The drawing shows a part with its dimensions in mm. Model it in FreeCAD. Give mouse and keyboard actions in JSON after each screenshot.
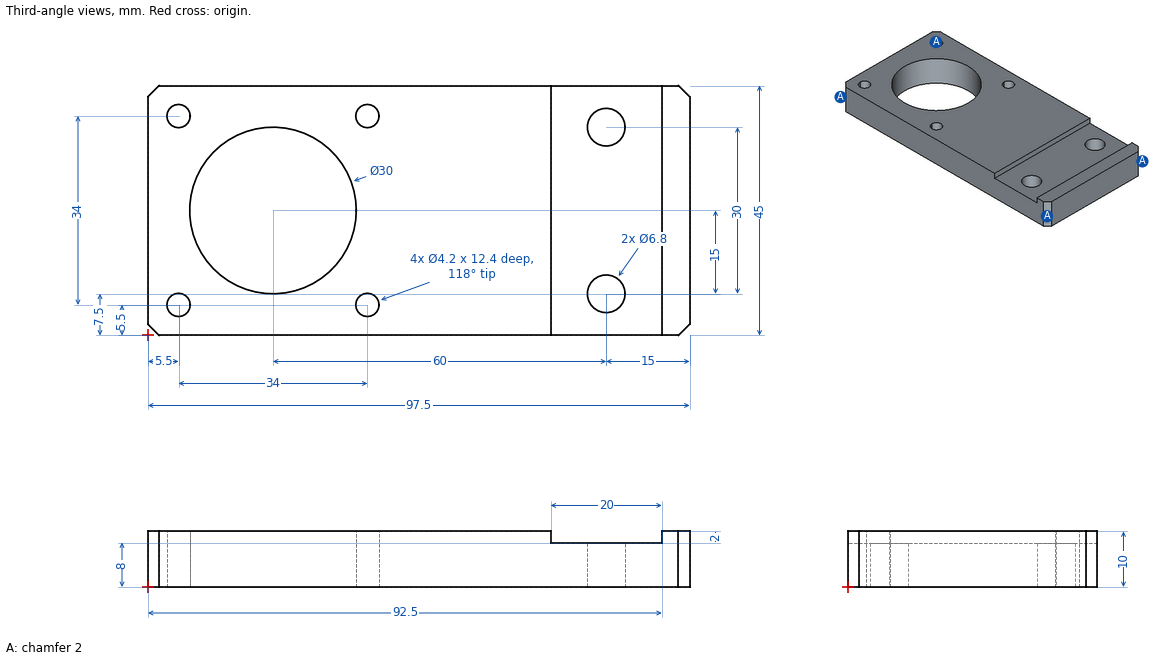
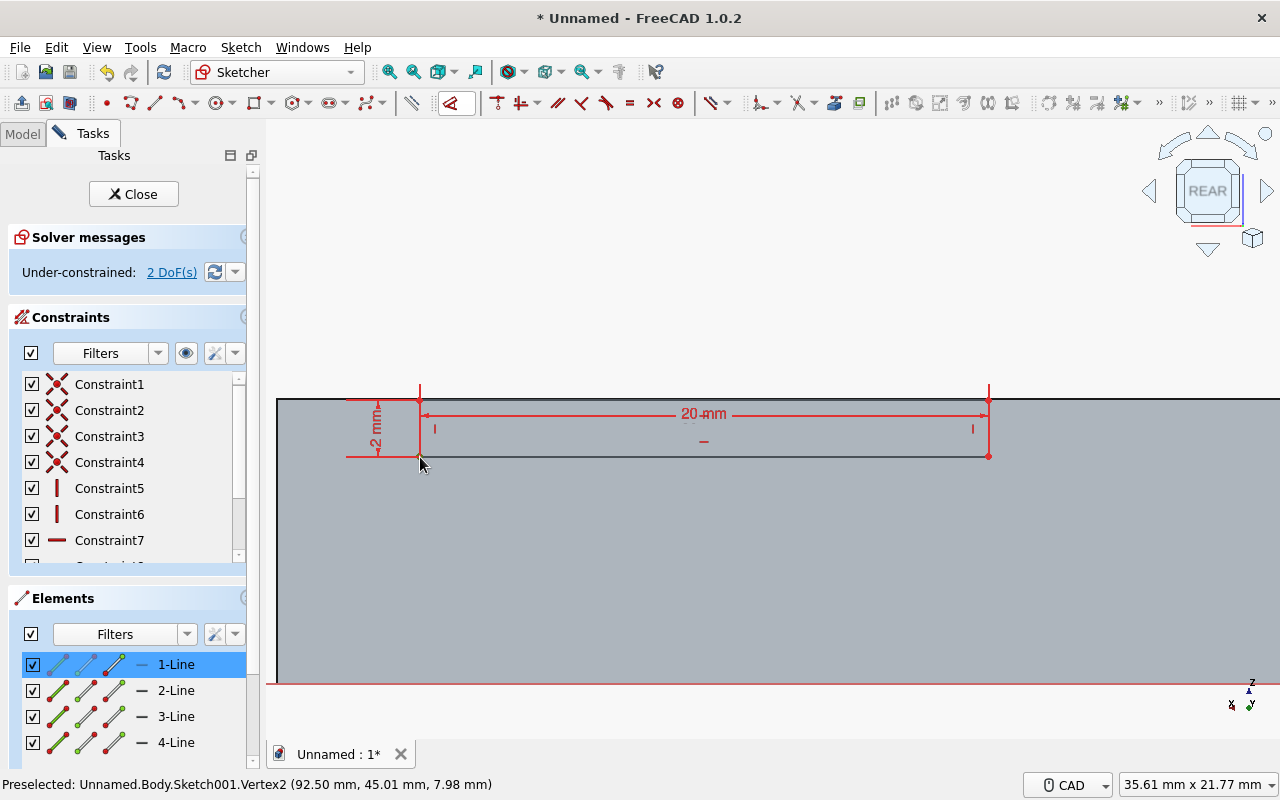
{"action": "key", "text": "i"}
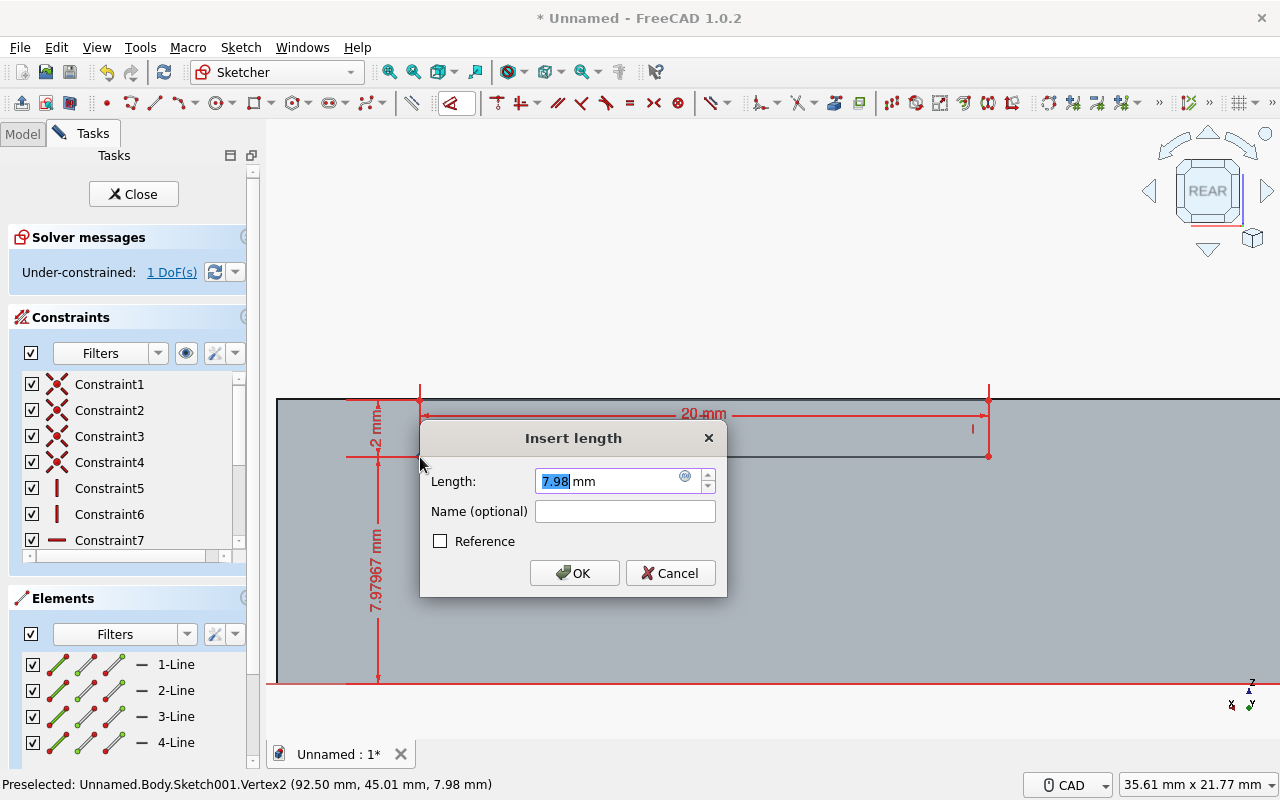
{"action": "type", "text": "8"}
{"action": "key", "text": "Return"}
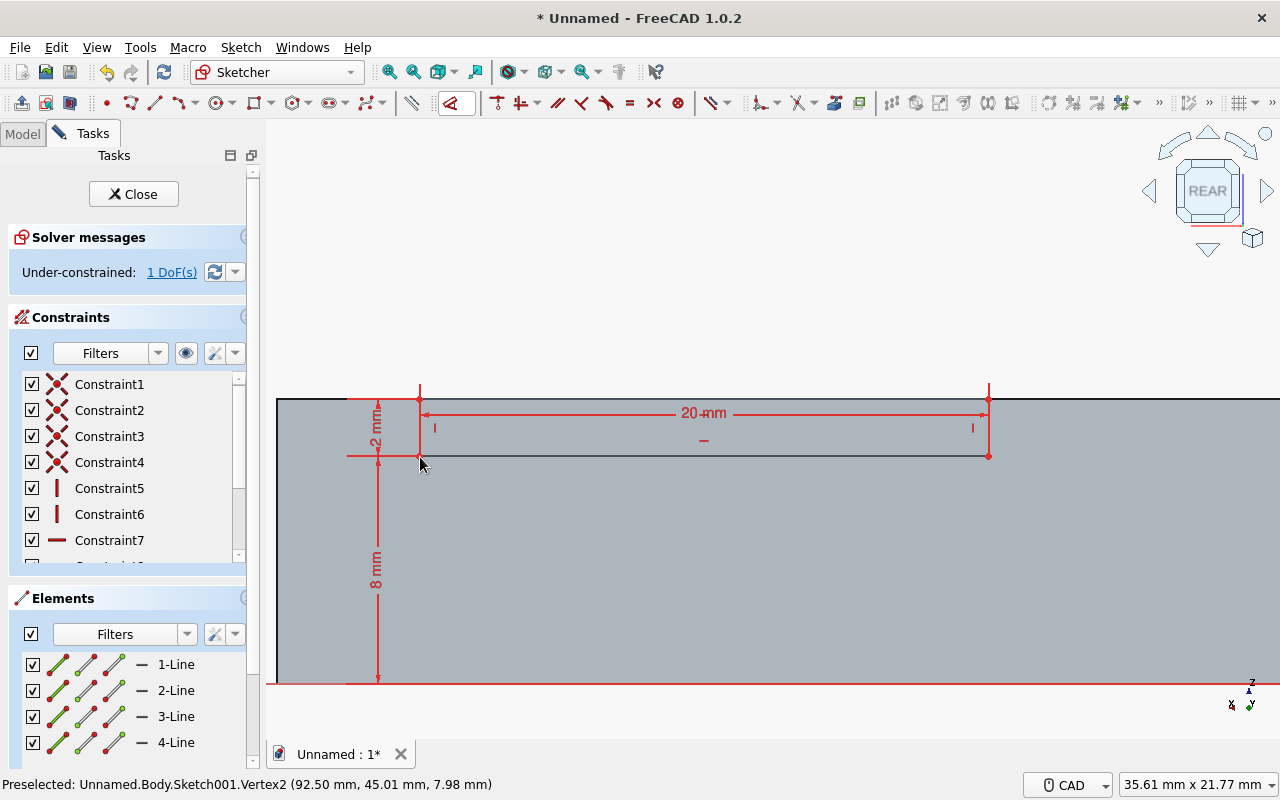
{"action": "left_click", "coordinate": [420, 399]}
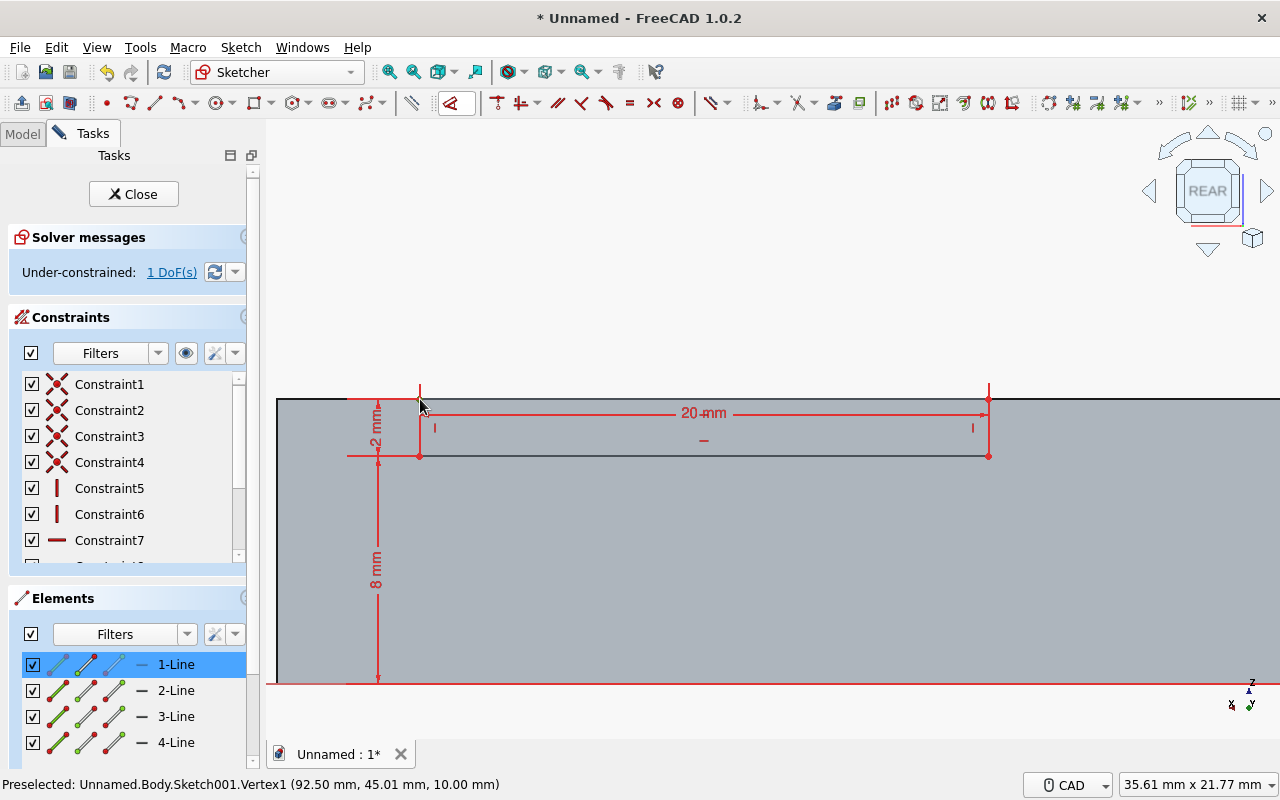
{"action": "left_click", "coordinate": [470, 104]}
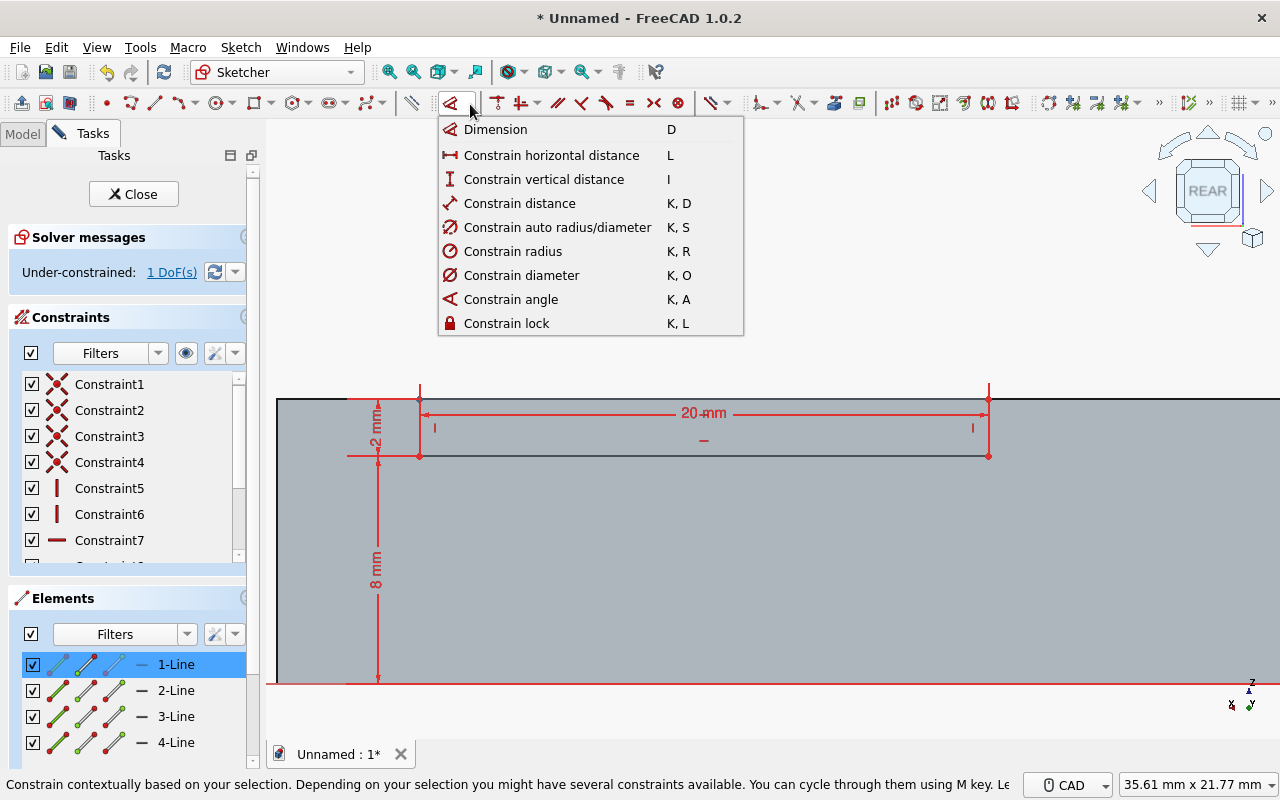
{"action": "left_click", "coordinate": [591, 155]}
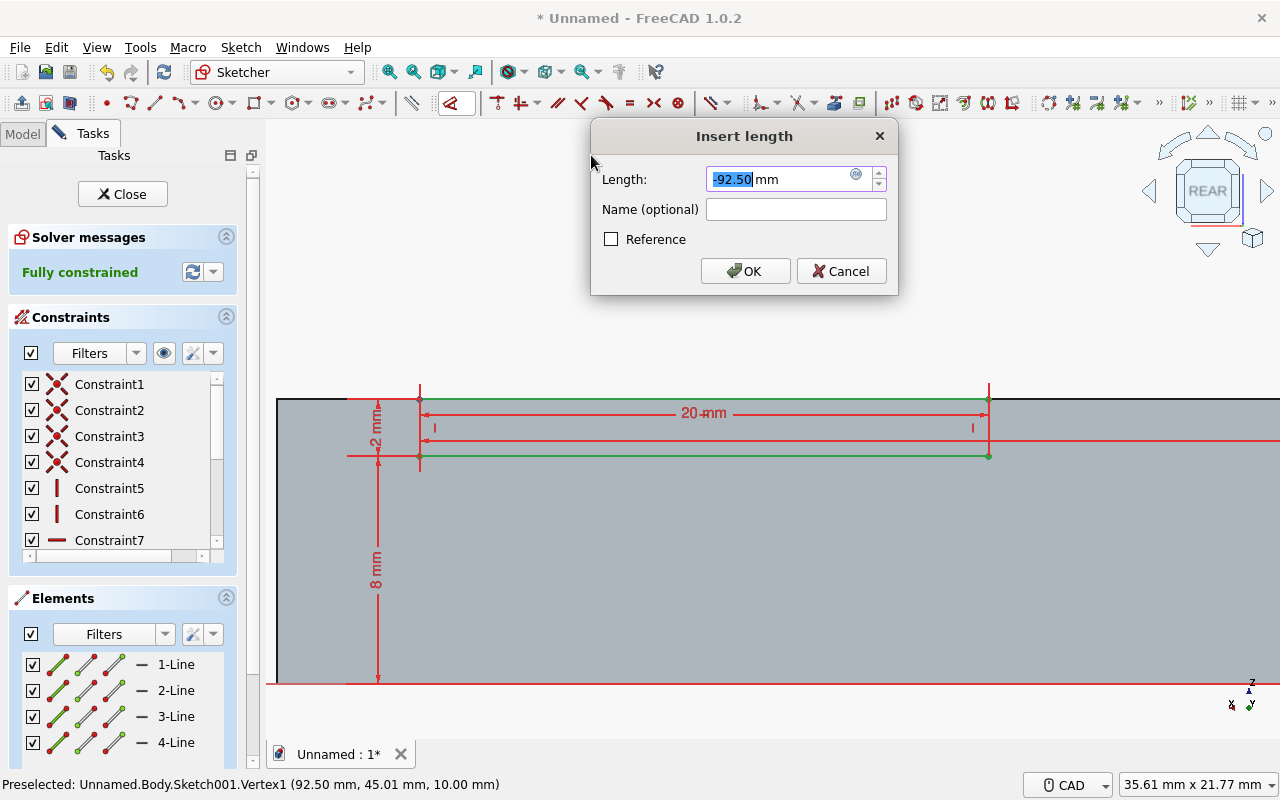
{"action": "type", "text": "-92.5"}
{"action": "key", "text": "Return"}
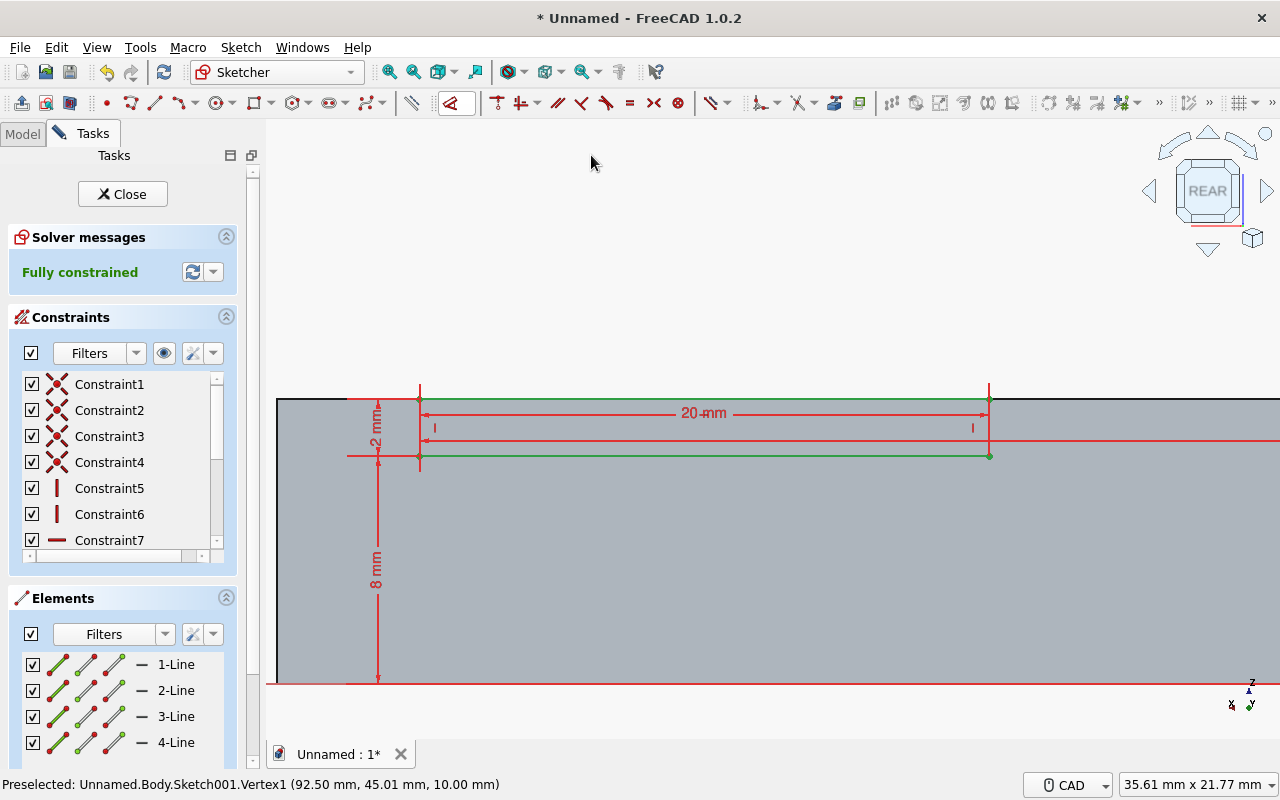
{"action": "left_click", "coordinate": [123, 194]}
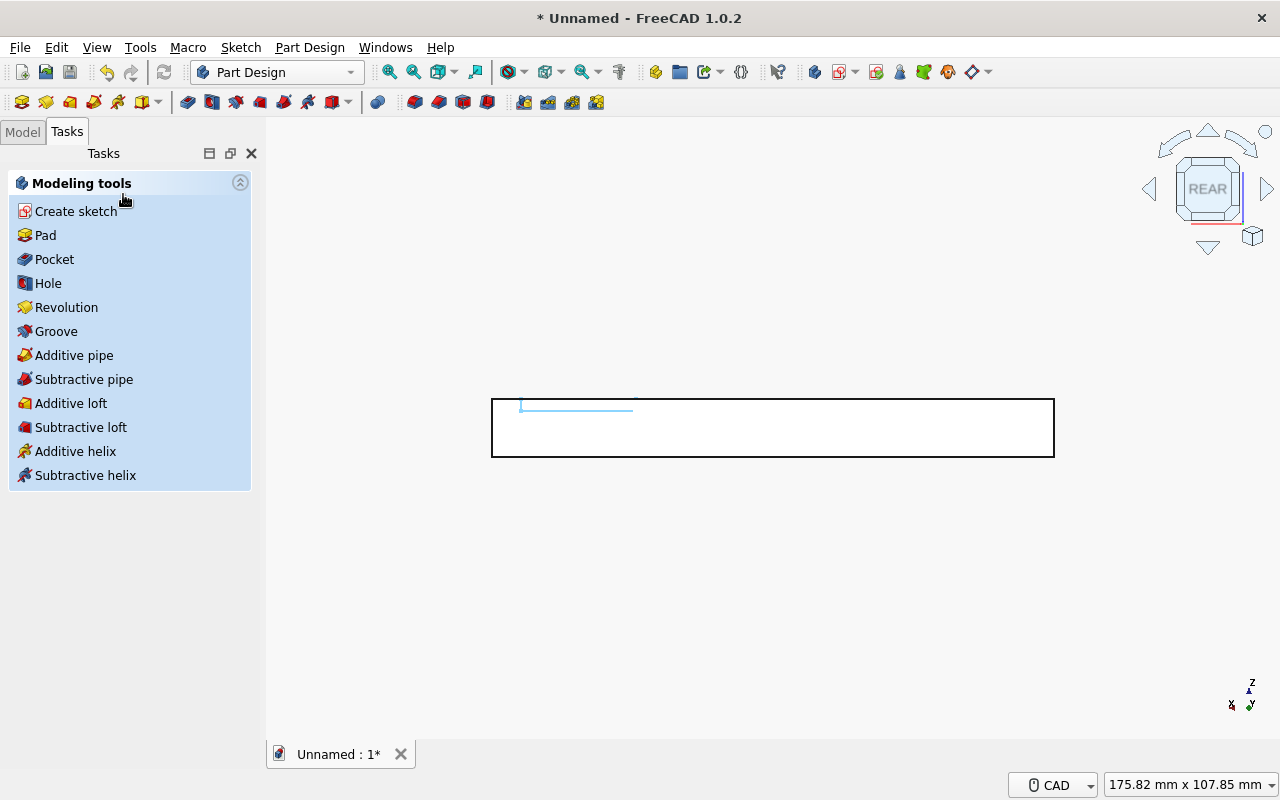
{"action": "left_click", "coordinate": [188, 102]}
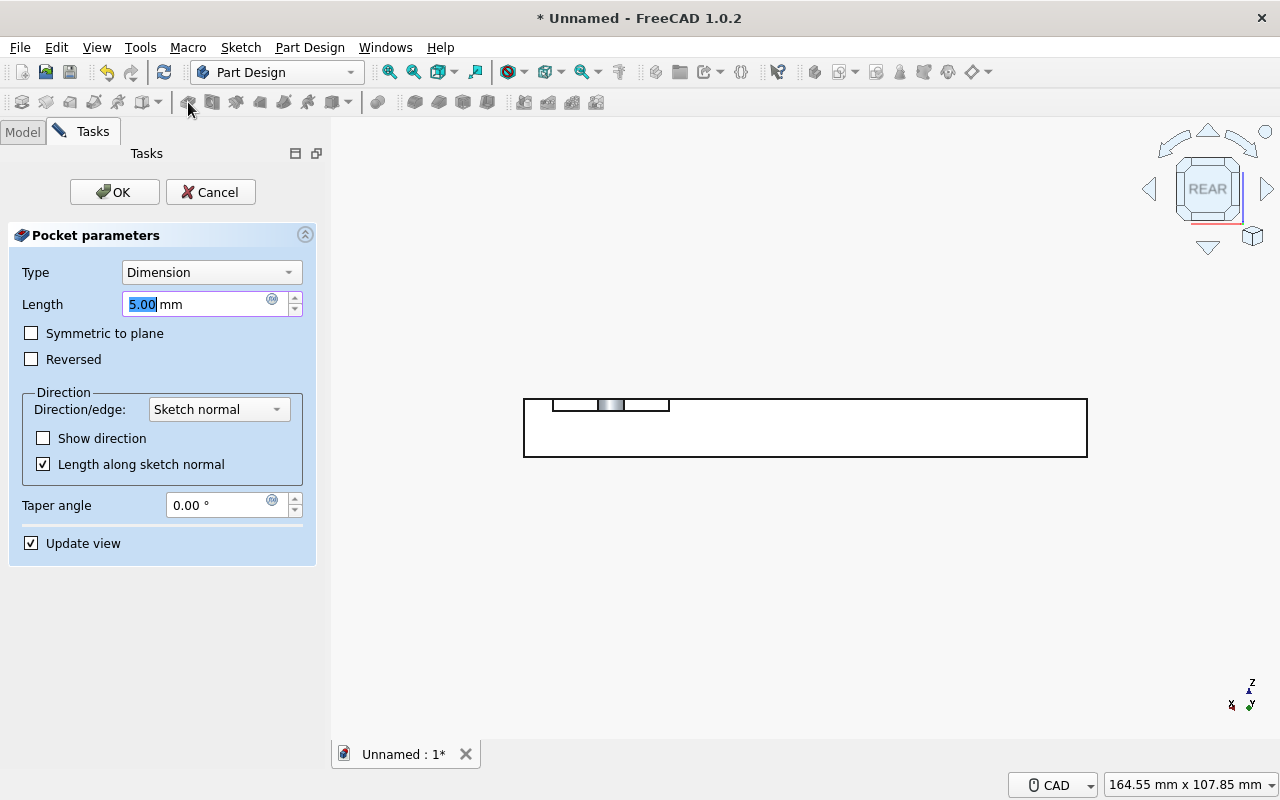
{"action": "left_click", "coordinate": [212, 272]}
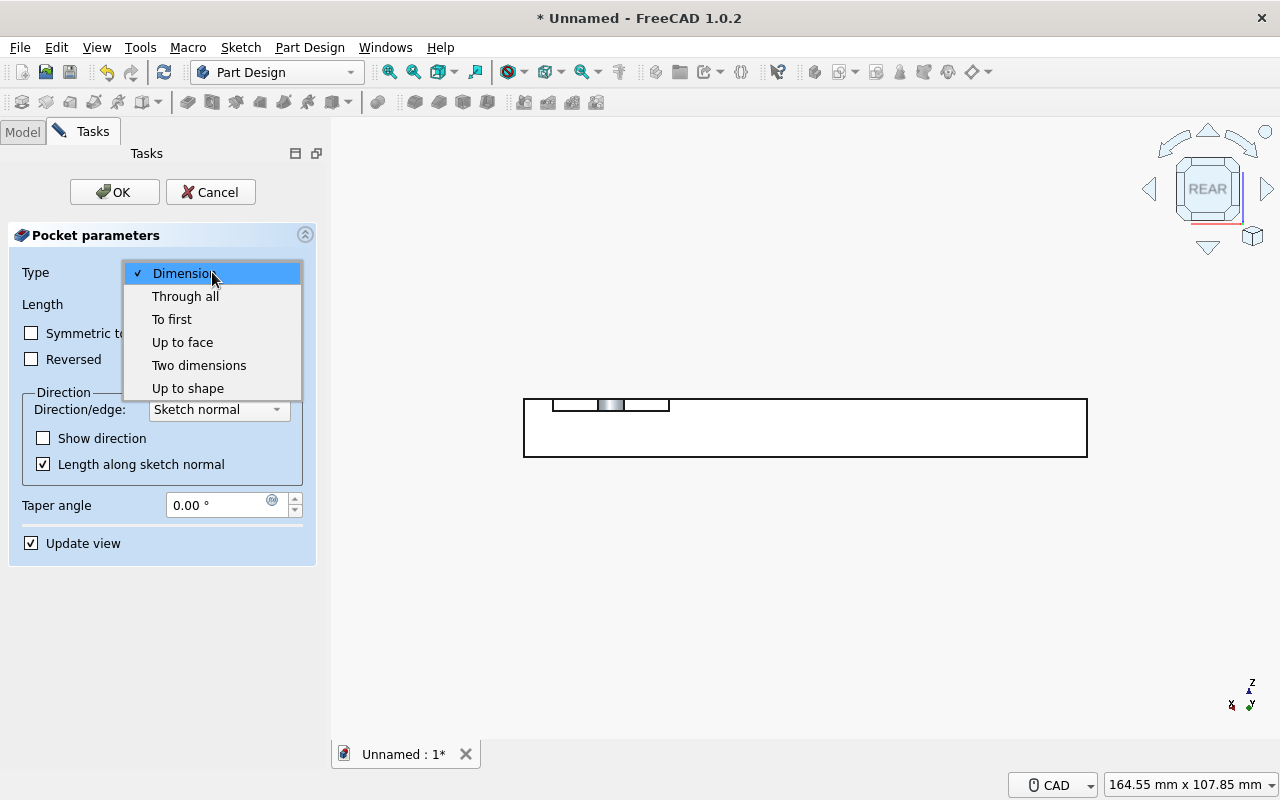
{"action": "left_click", "coordinate": [212, 320]}